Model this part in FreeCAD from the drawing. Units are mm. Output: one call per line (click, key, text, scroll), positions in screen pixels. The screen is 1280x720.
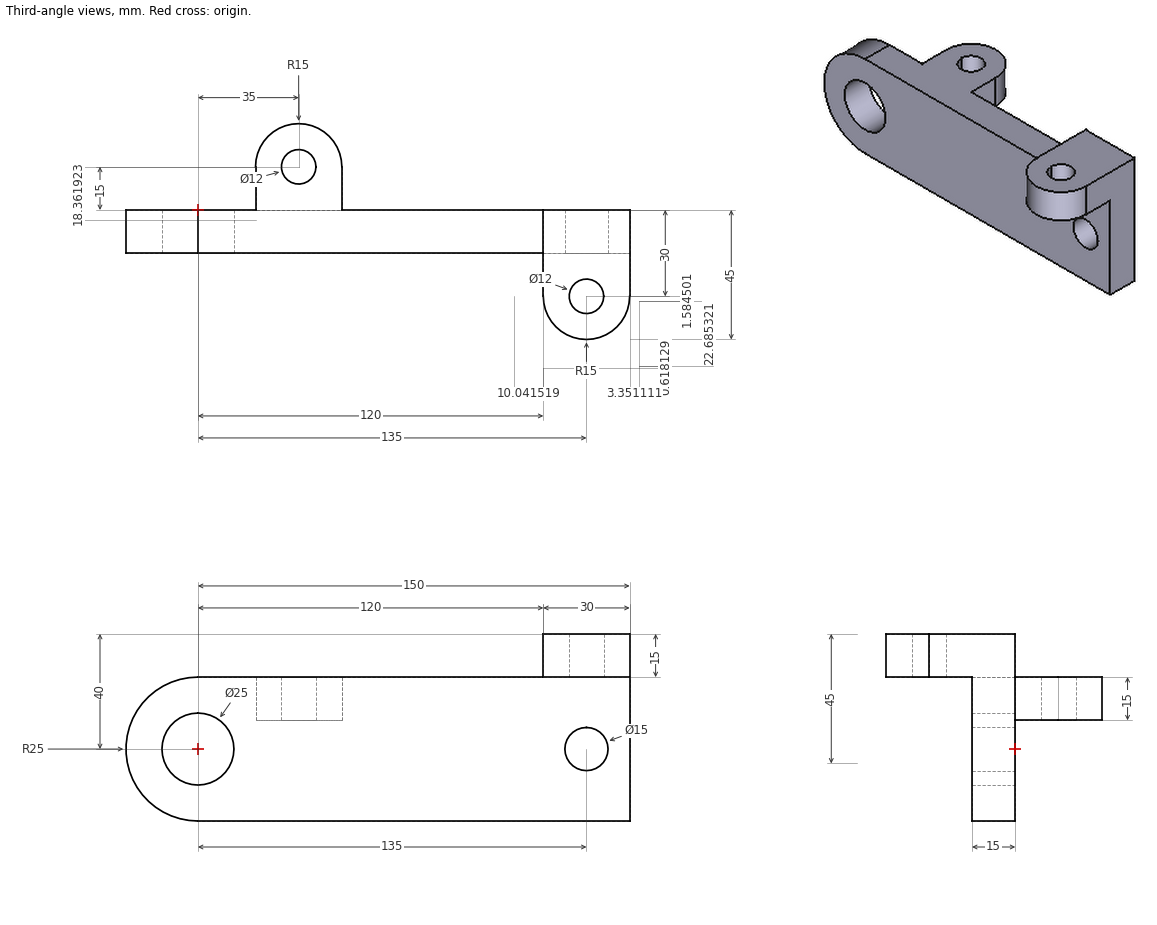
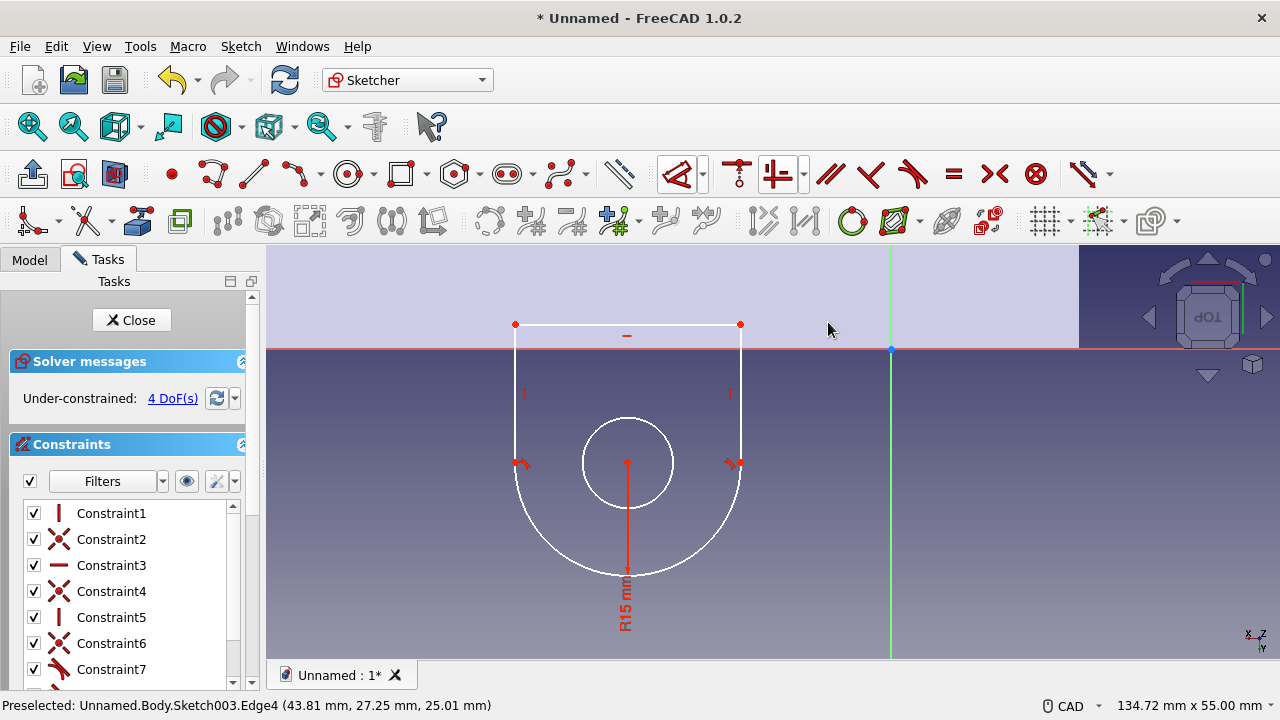
click(660, 431)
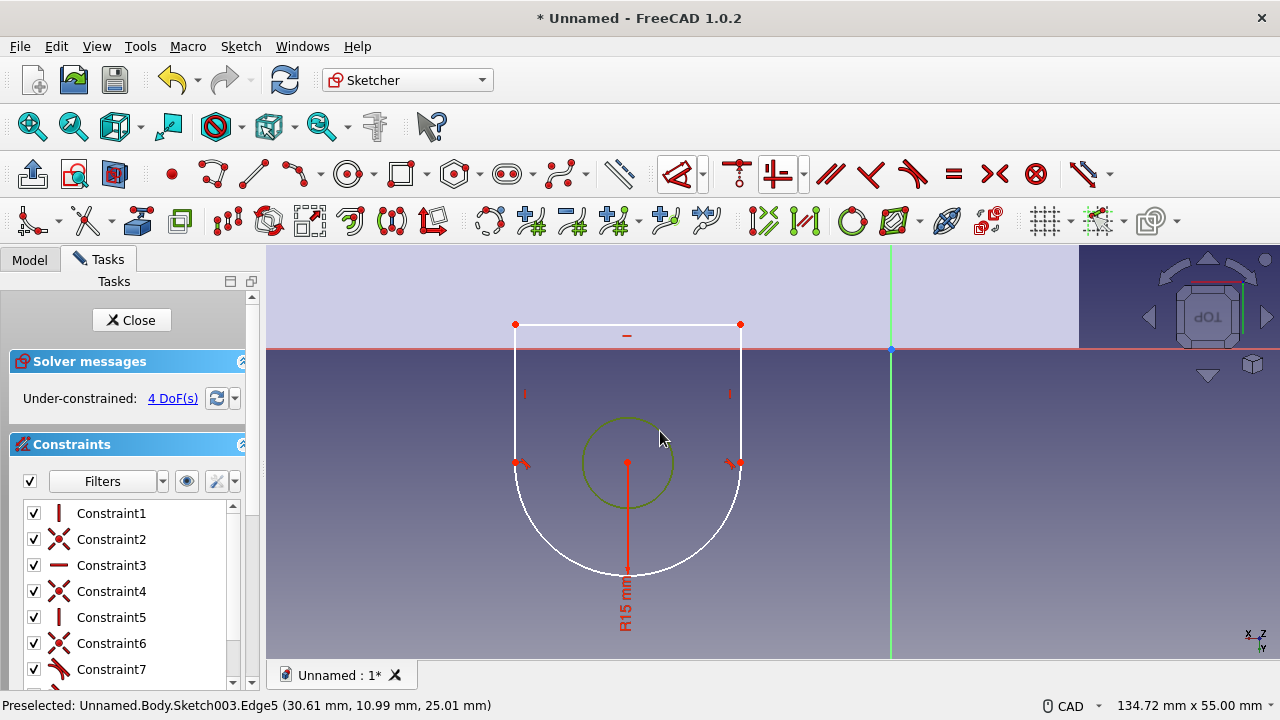
click(702, 174)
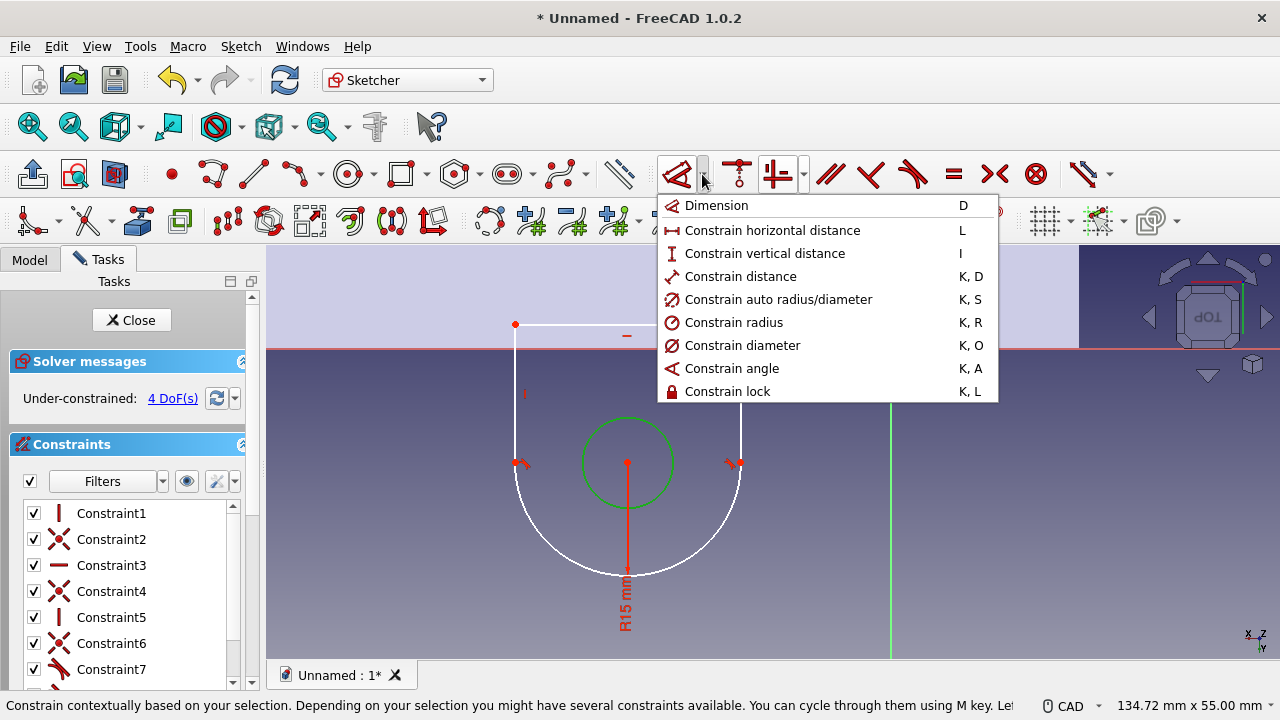
click(828, 346)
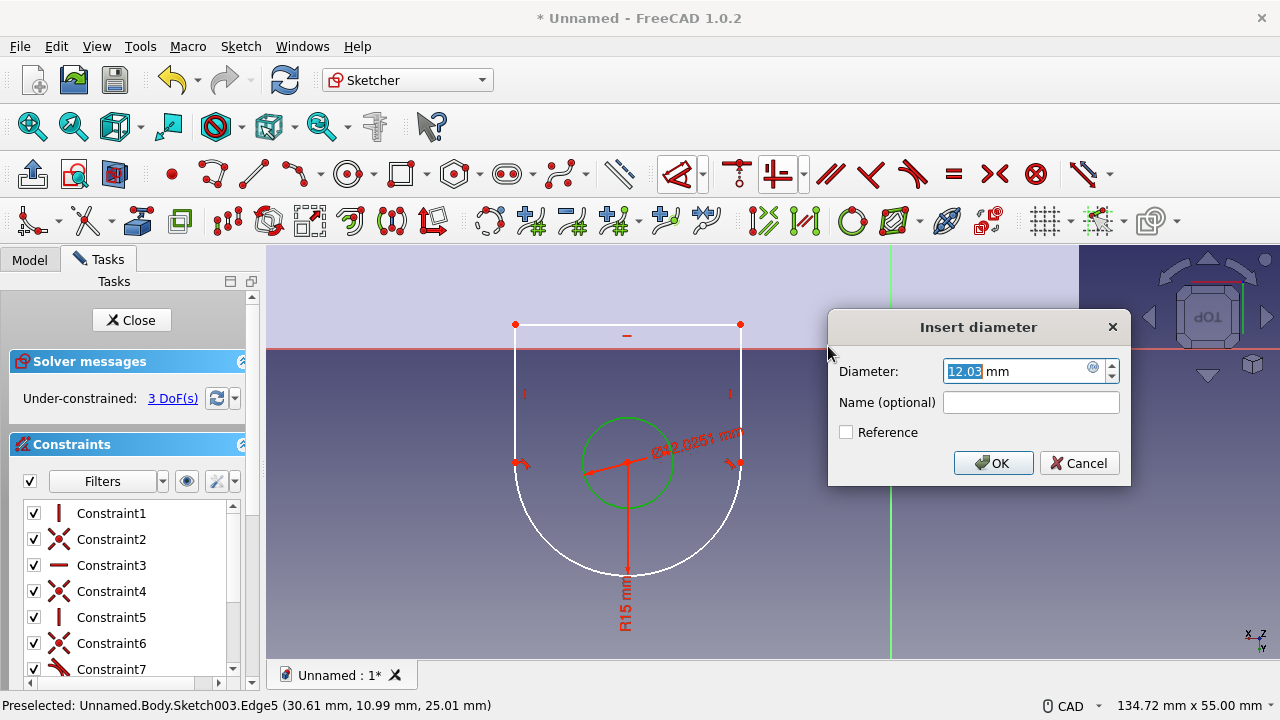
text(12)
key(Return)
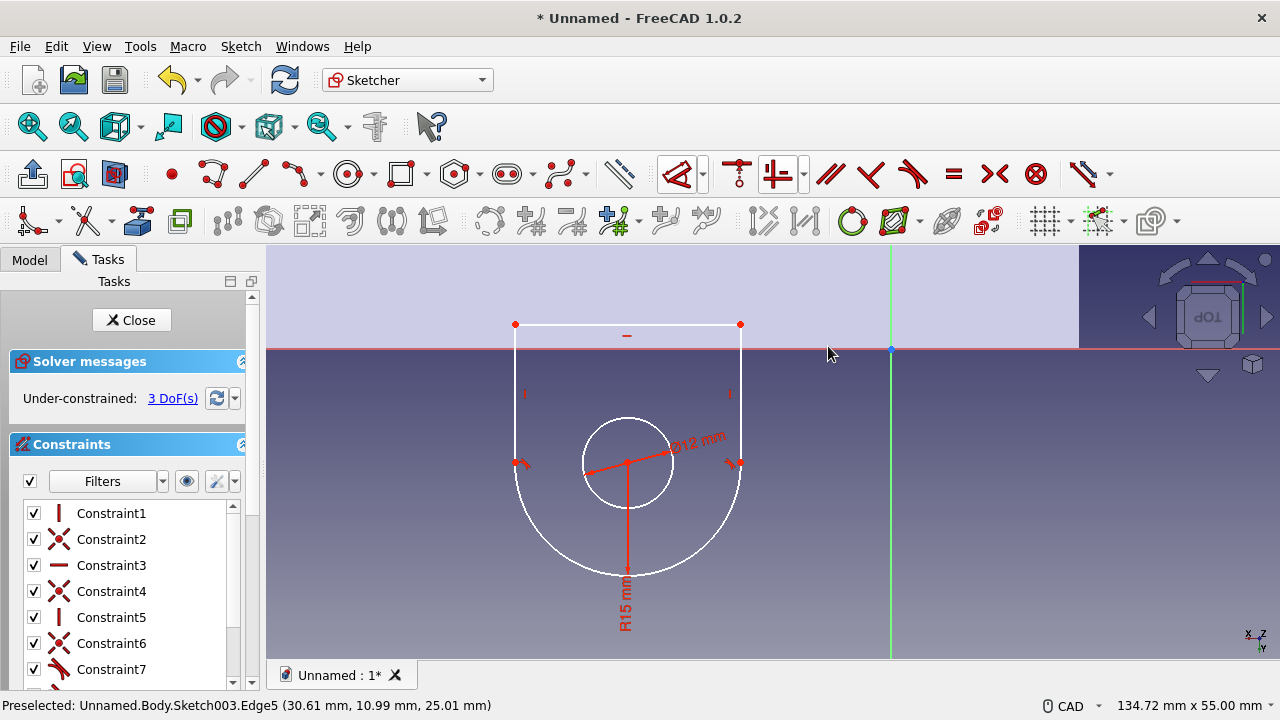
click(628, 463)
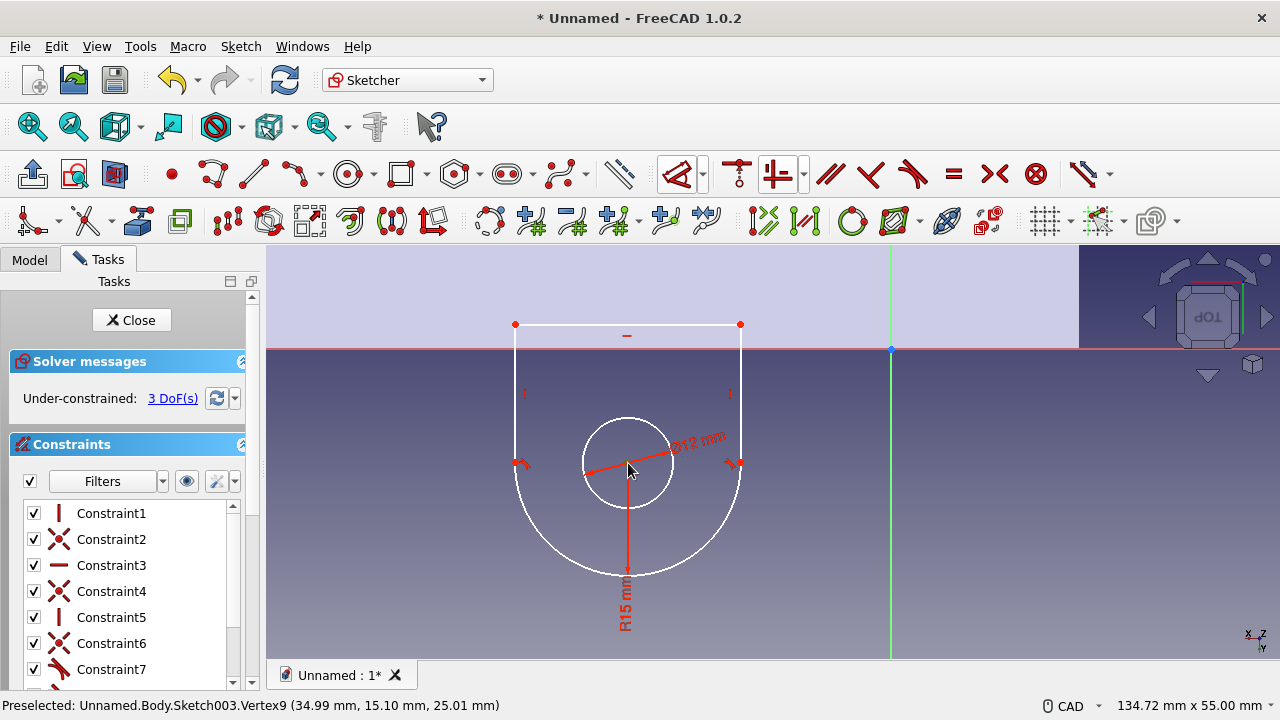
key(l)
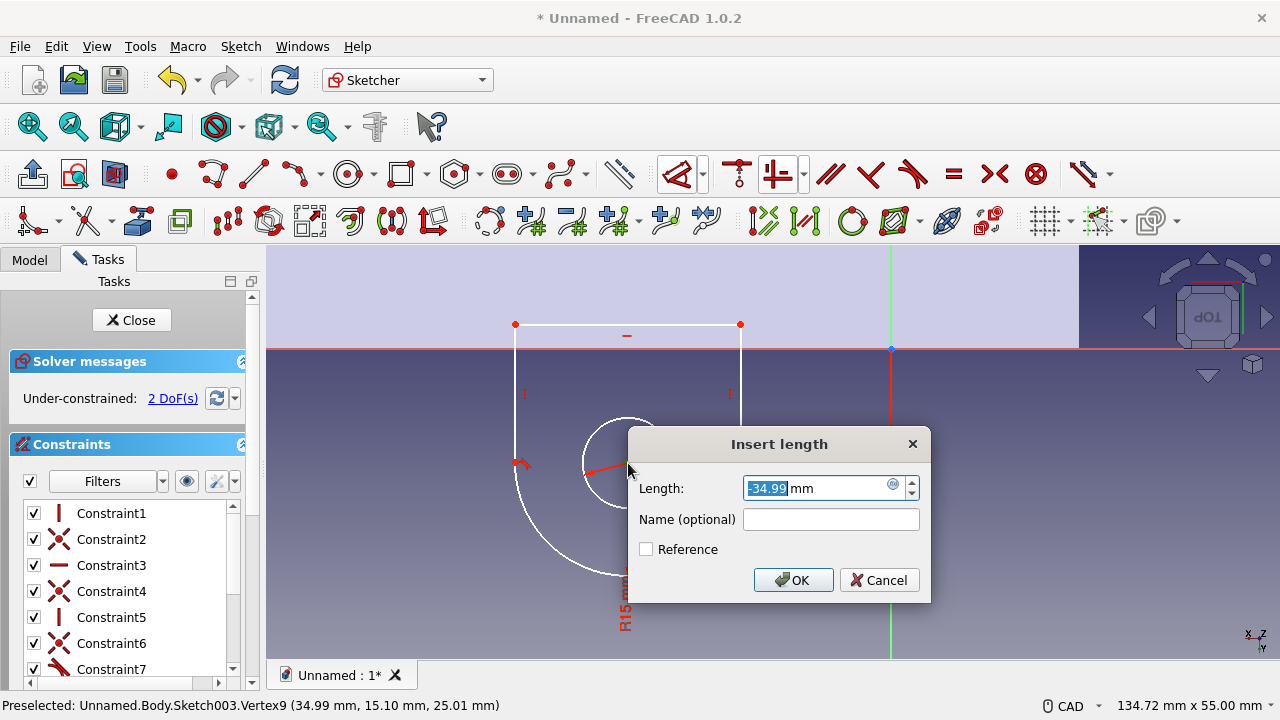
text(-35)
key(Return)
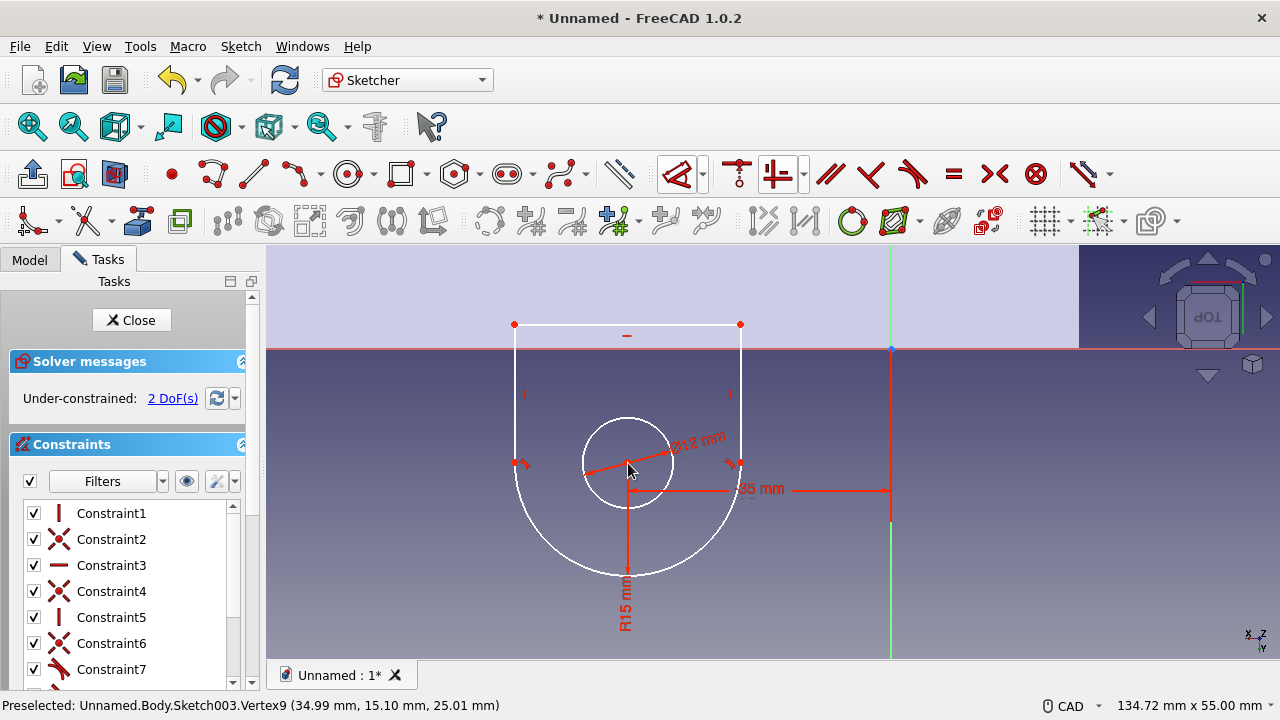
click(628, 463)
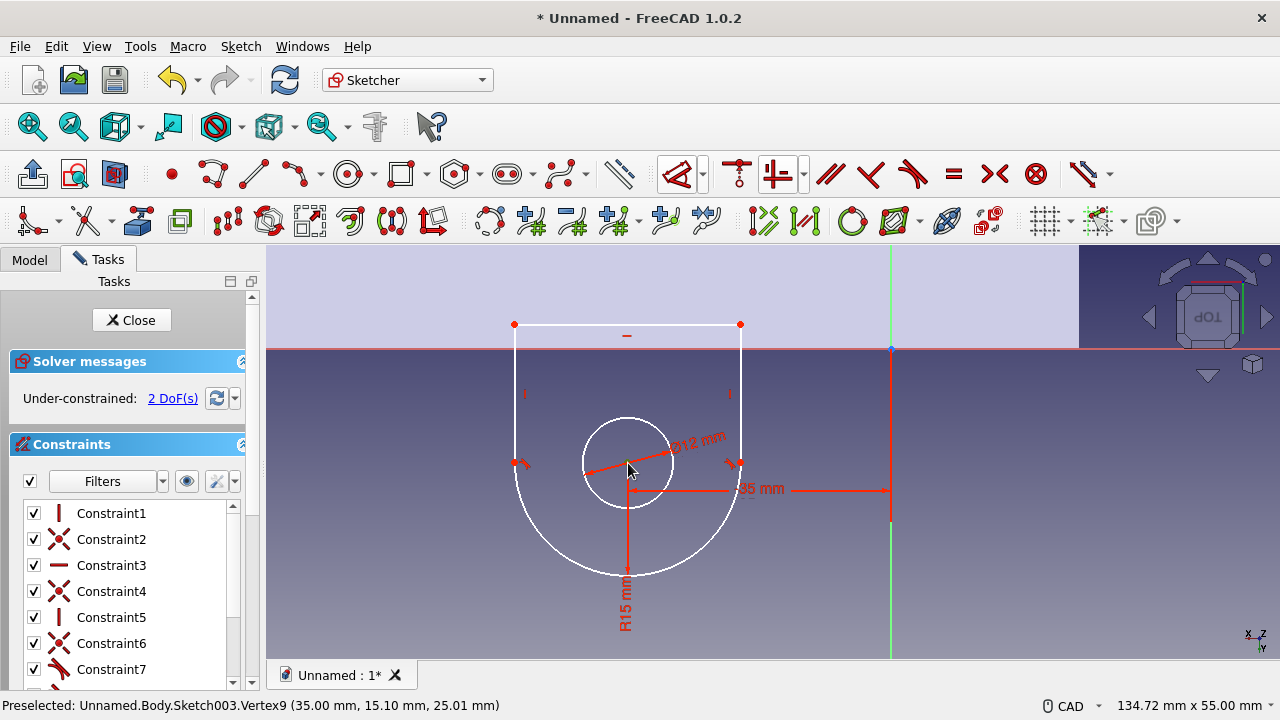
key(i)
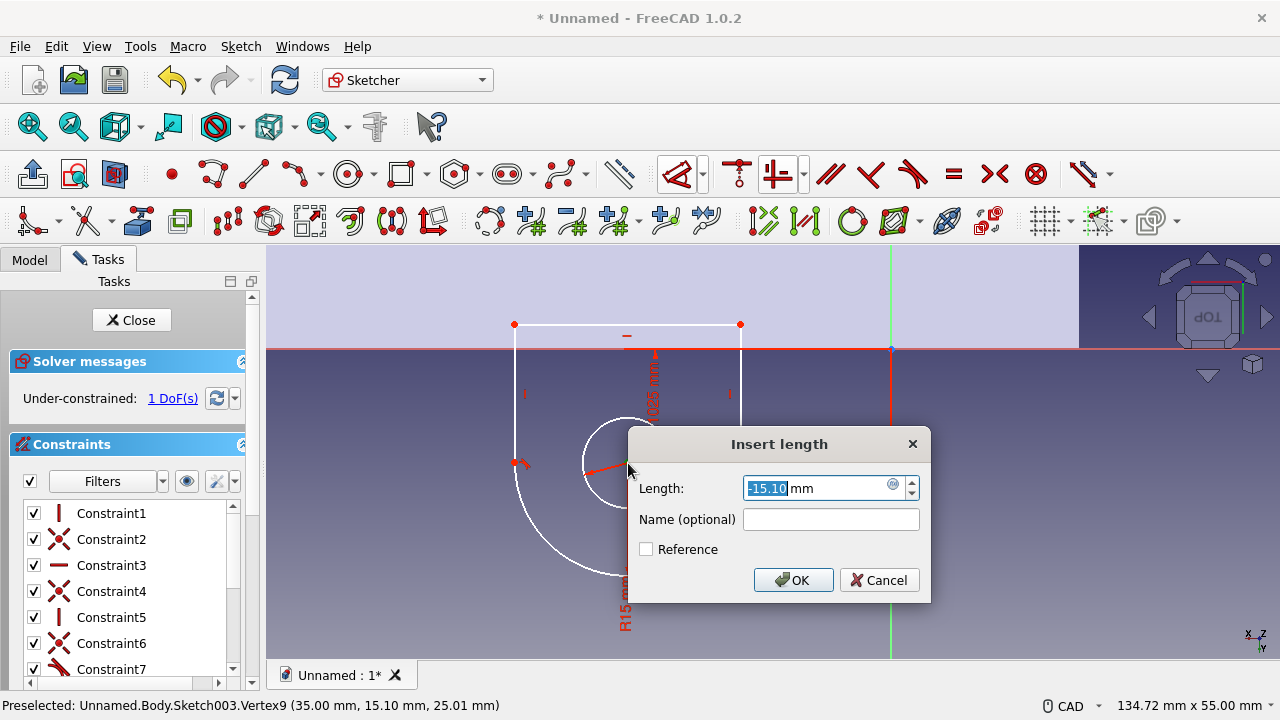
text(-15)
key(Return)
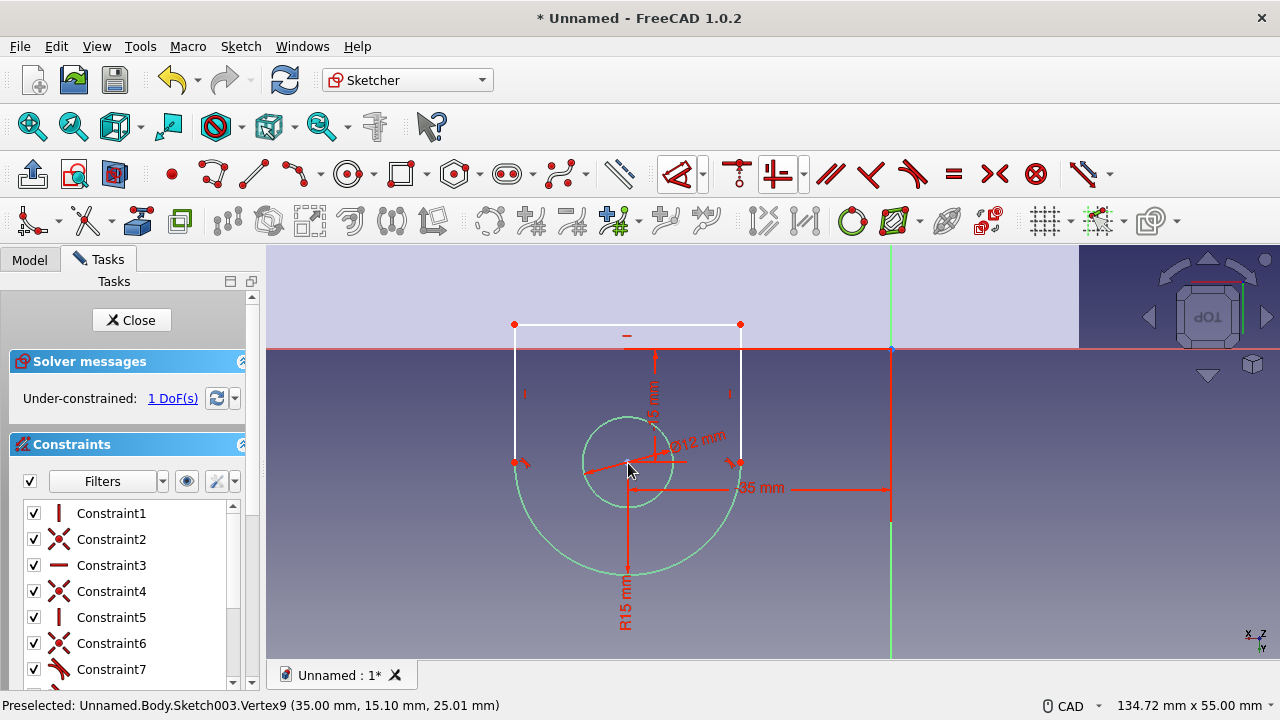
click(741, 421)